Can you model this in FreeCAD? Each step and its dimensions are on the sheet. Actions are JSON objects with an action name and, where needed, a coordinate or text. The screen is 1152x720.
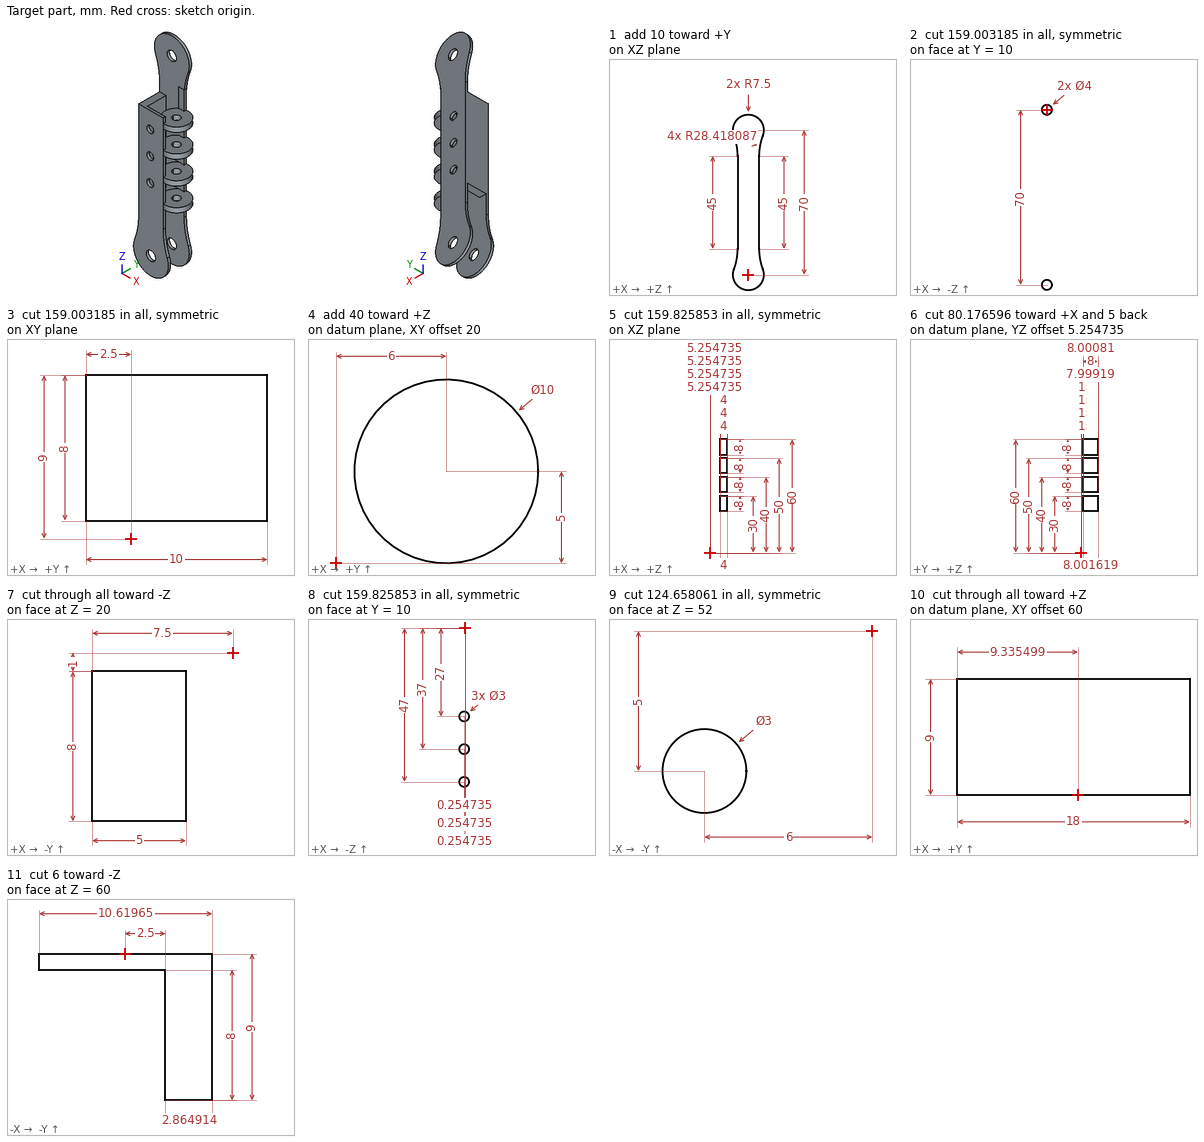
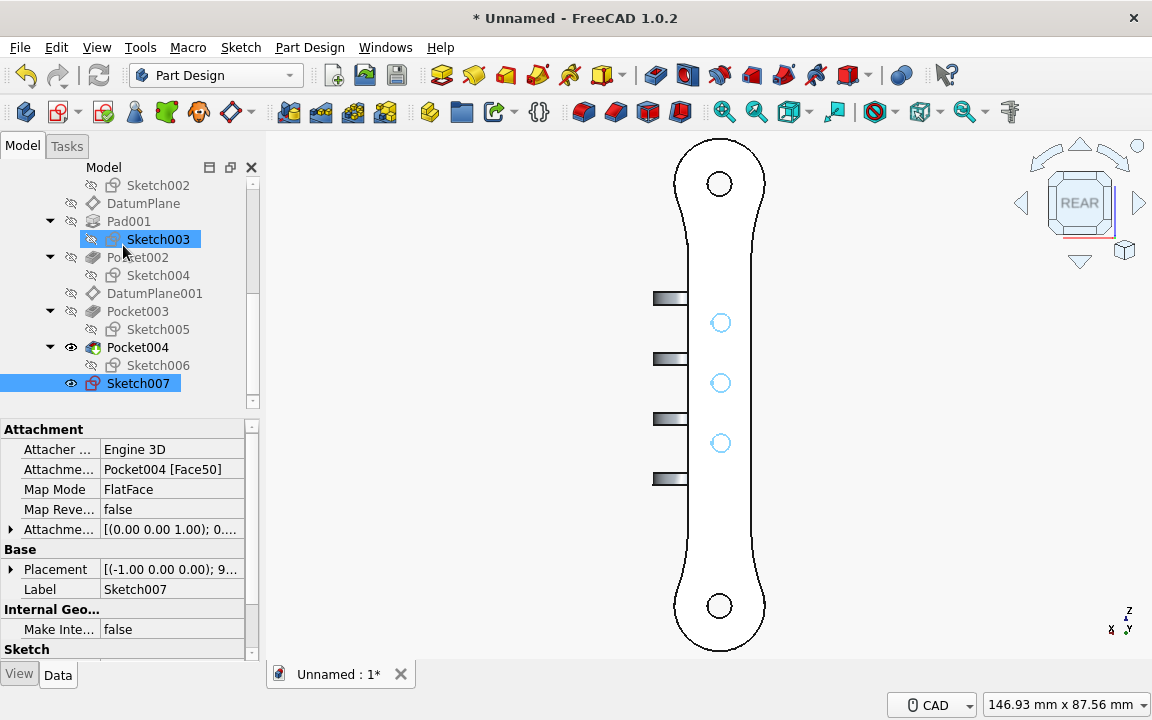
{"action": "left_click", "coordinate": [656, 76]}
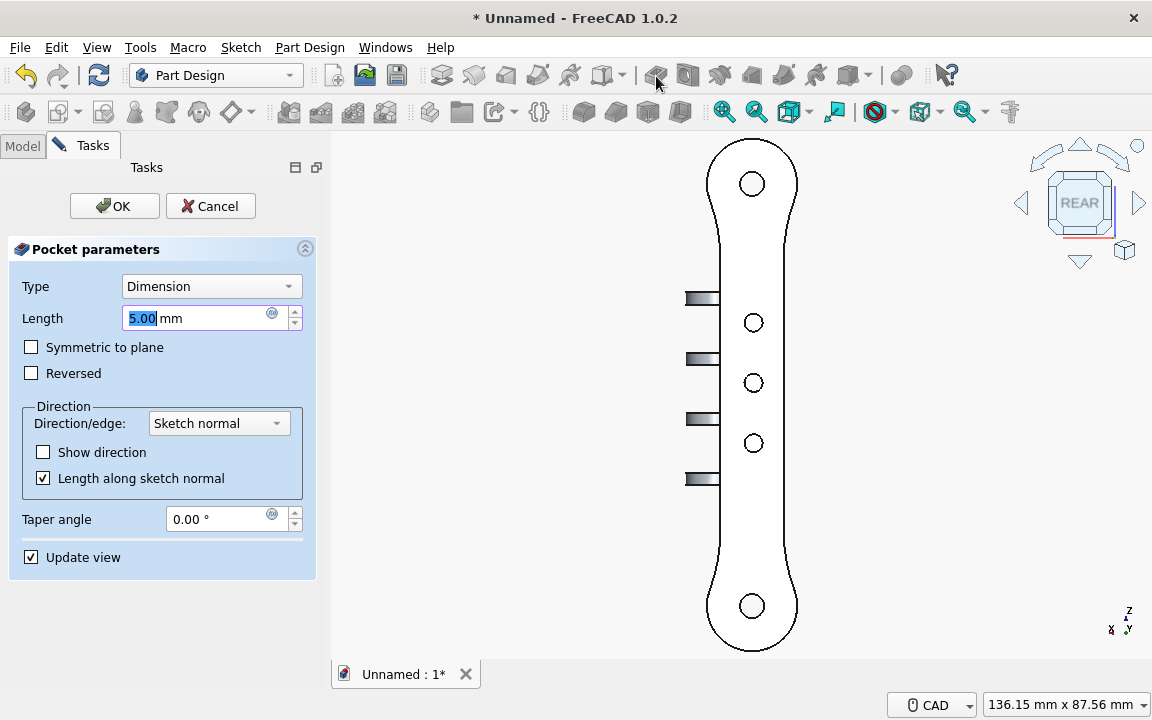
{"action": "type", "text": "159.825853"}
{"action": "key", "text": "Tab"}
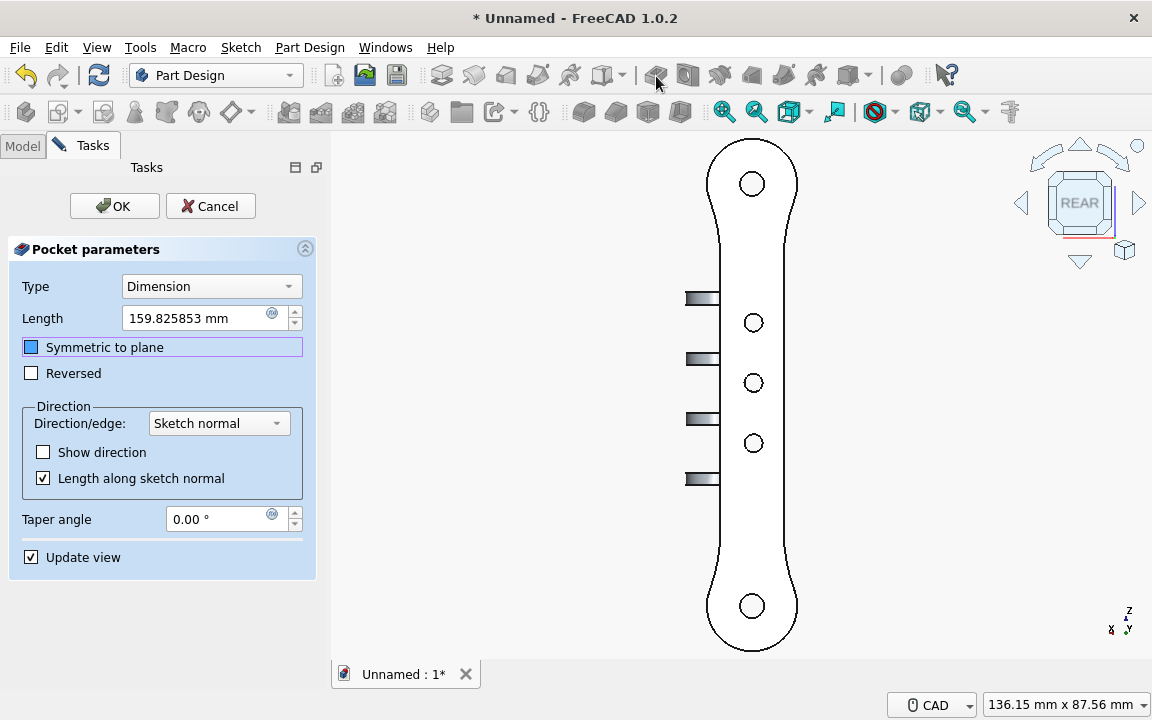
{"action": "left_click", "coordinate": [30, 347]}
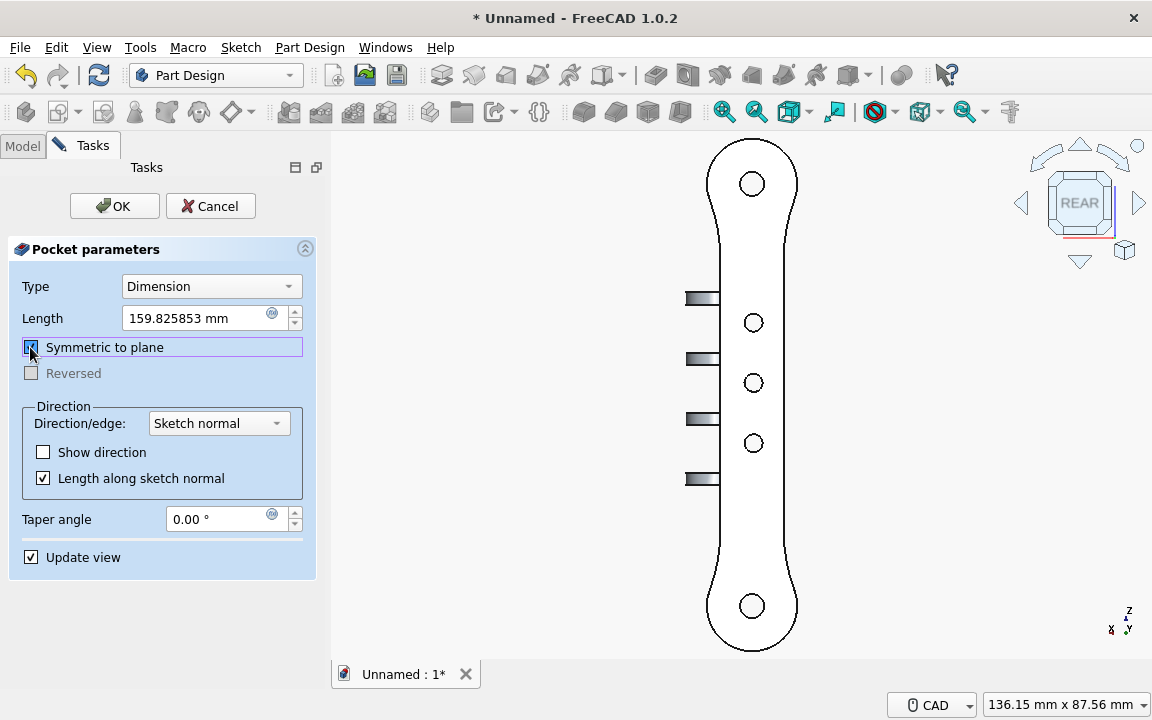
{"action": "left_click", "coordinate": [115, 206]}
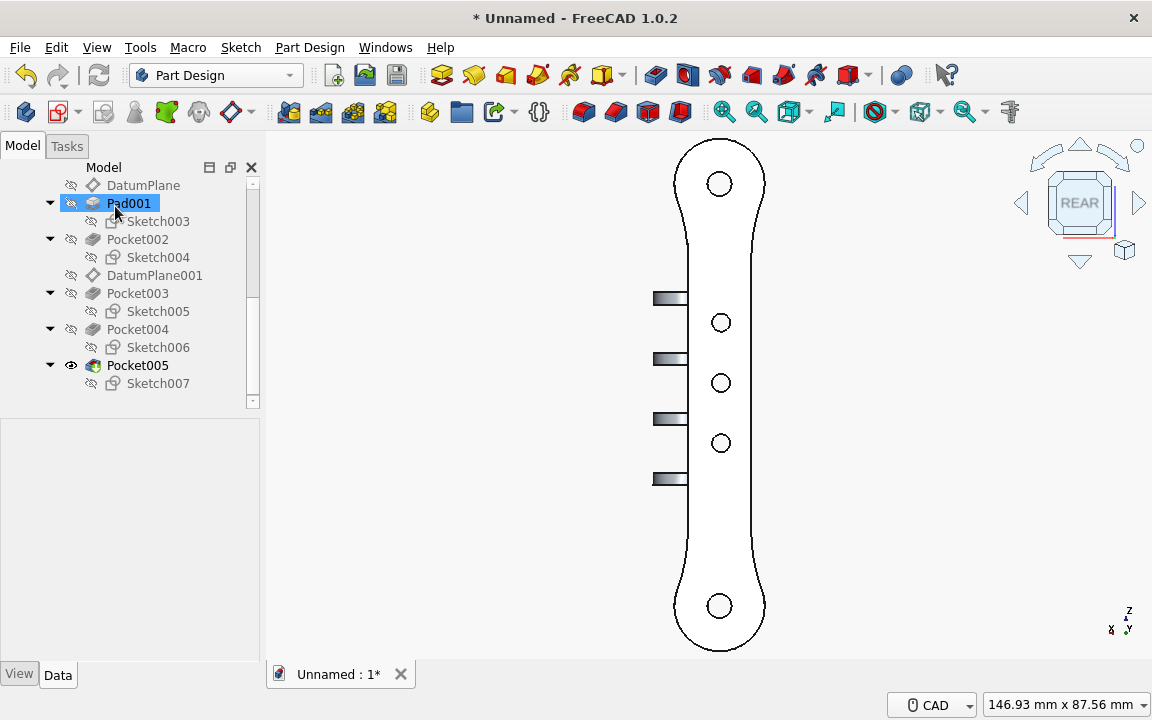
{"action": "key", "text": "0"}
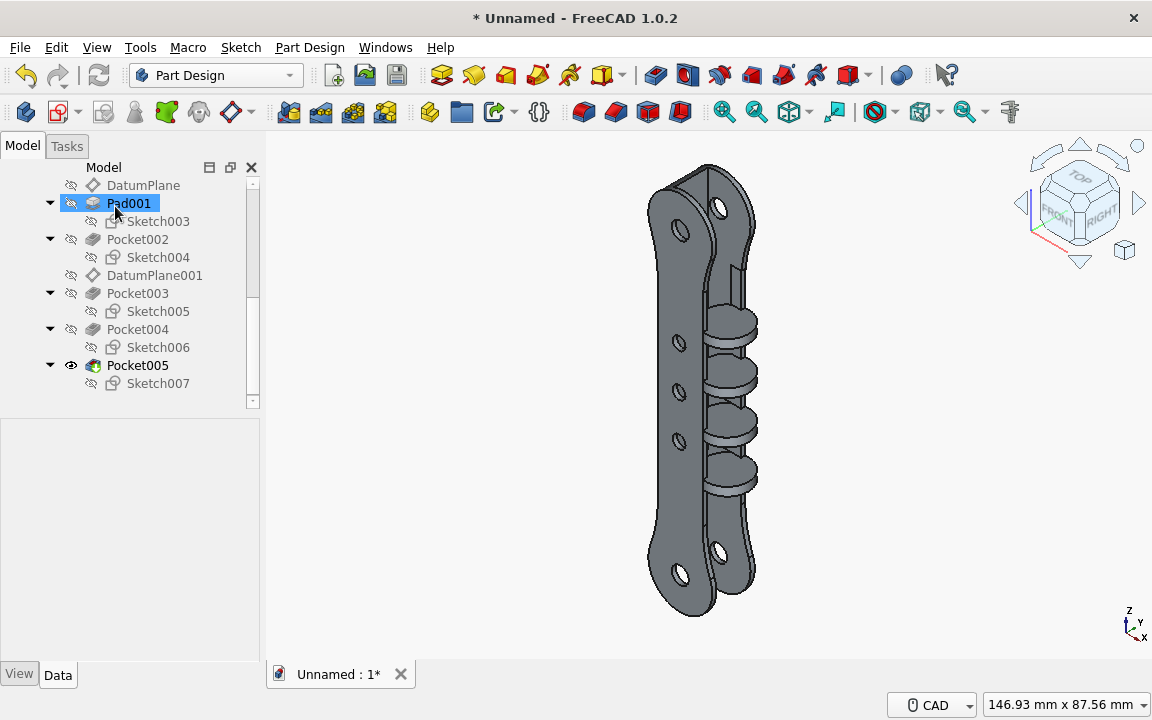
{"action": "left_click", "coordinate": [727, 321]}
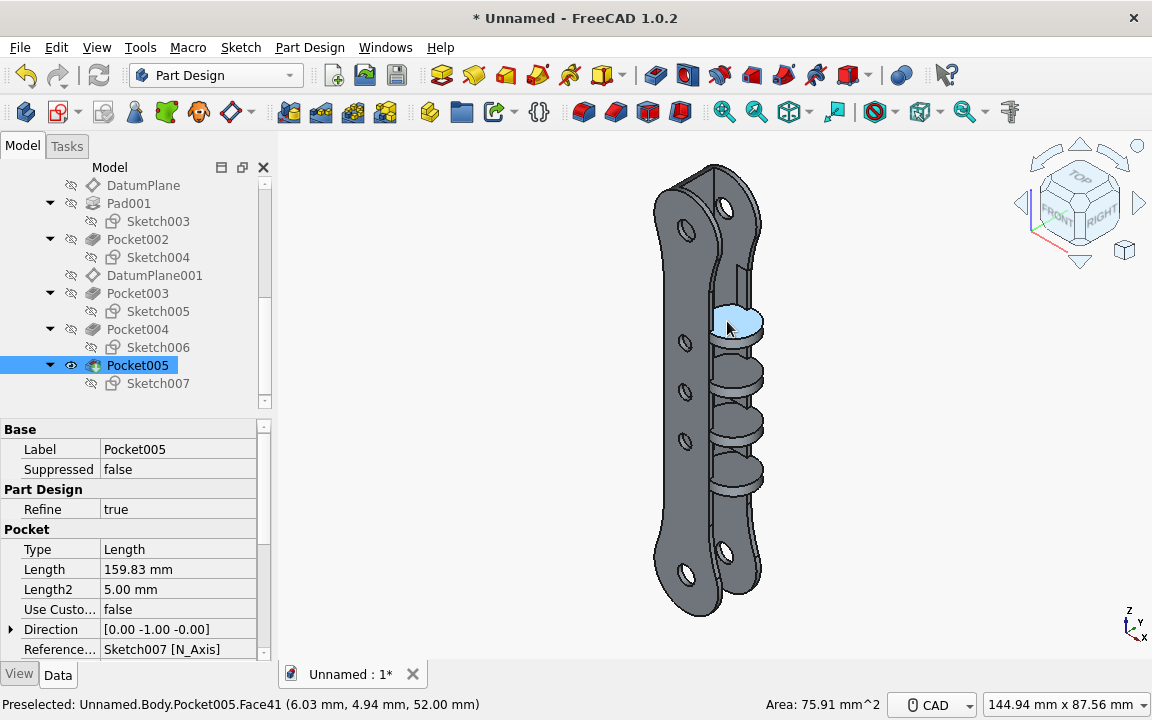
{"action": "left_click", "coordinate": [58, 112]}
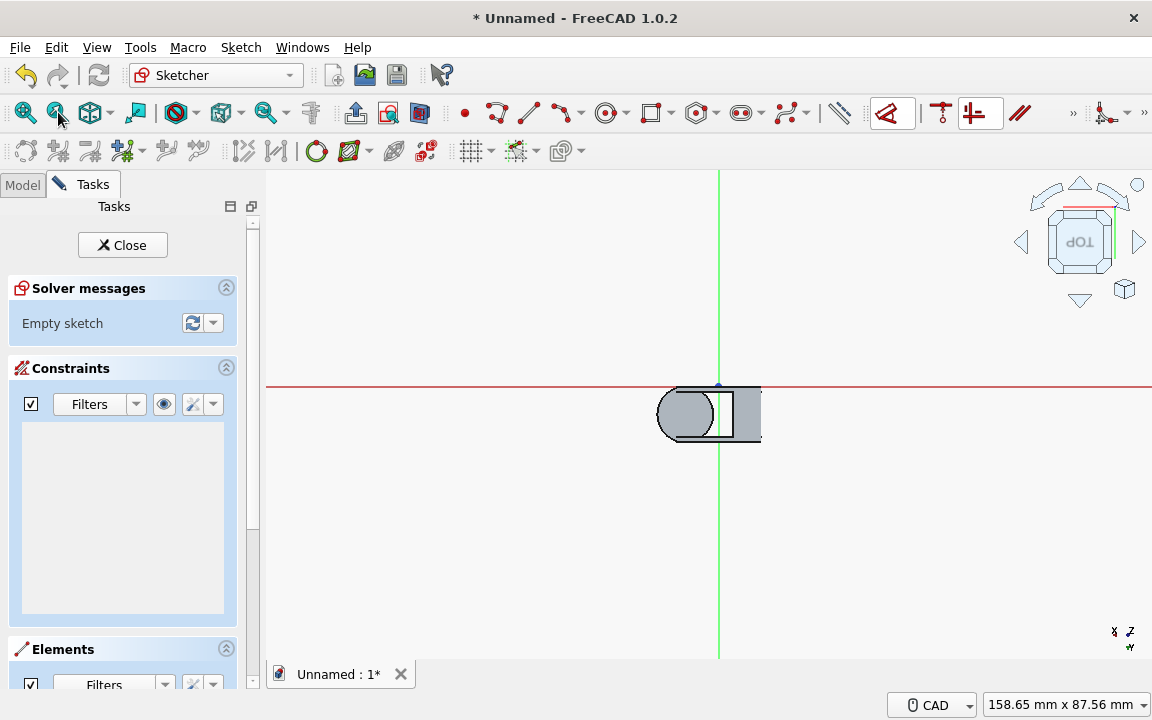
{"action": "scroll", "coordinate": [688, 415], "scroll_direction": "up", "scroll_amount": 15}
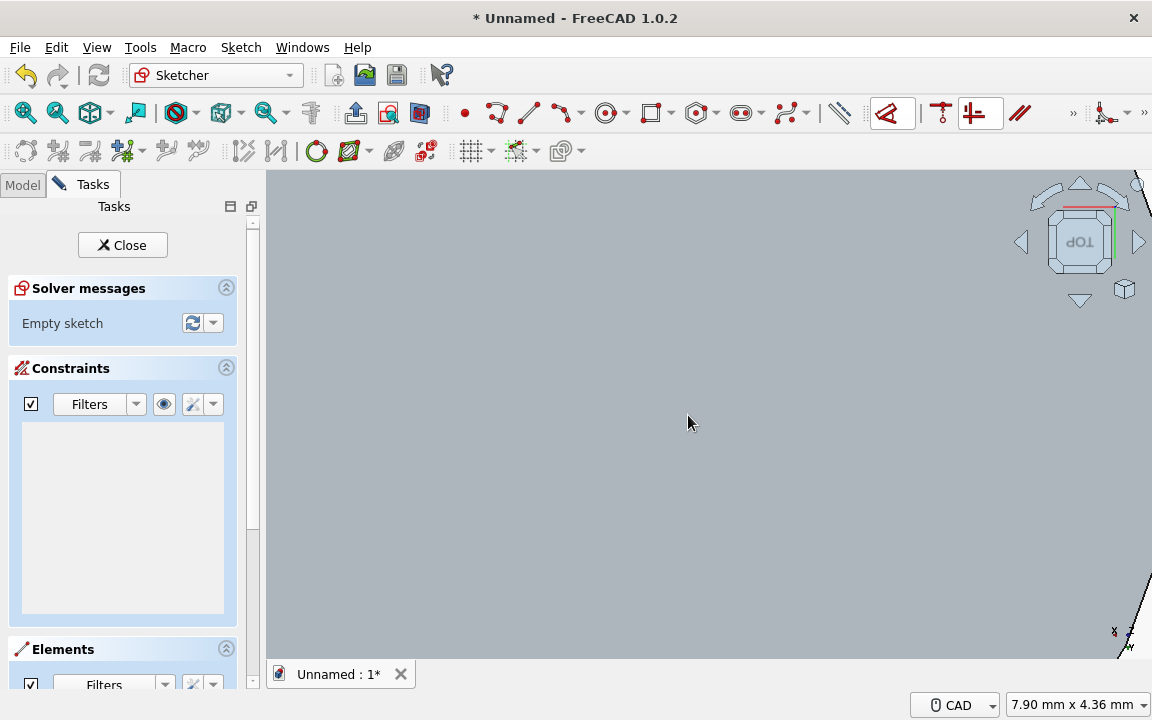
{"action": "left_click", "coordinate": [606, 114]}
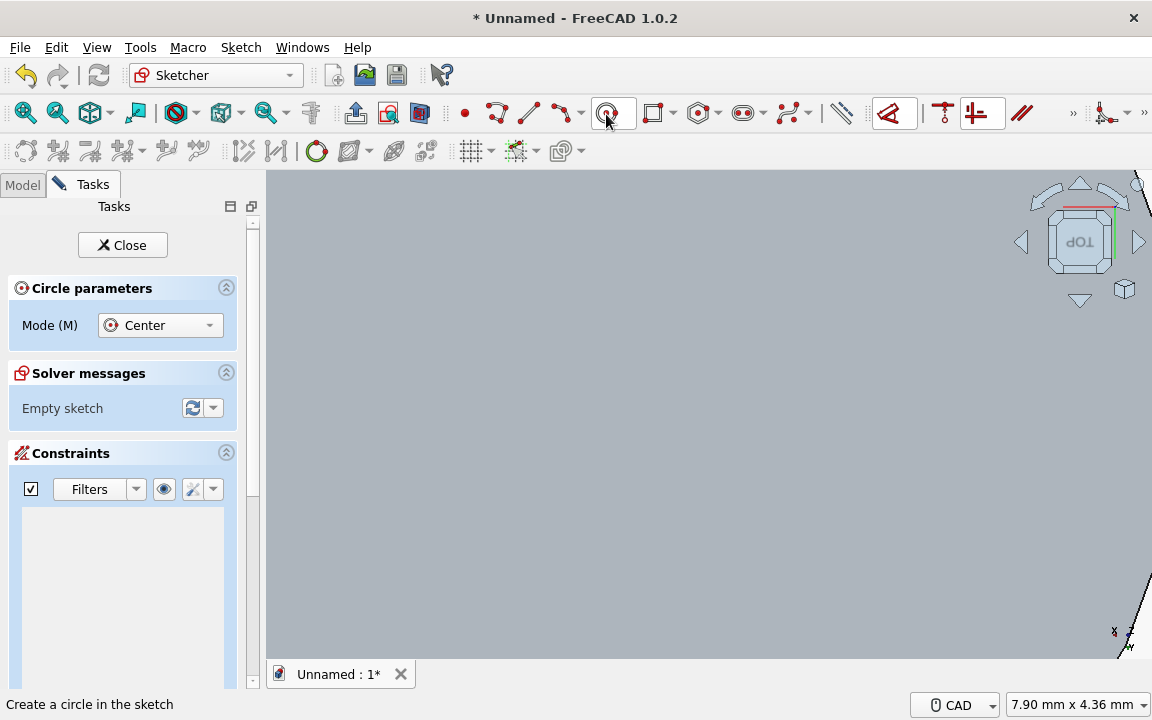
{"action": "left_click", "coordinate": [624, 395]}
{"action": "left_click", "coordinate": [743, 276]}
{"action": "key", "text": "Escape"}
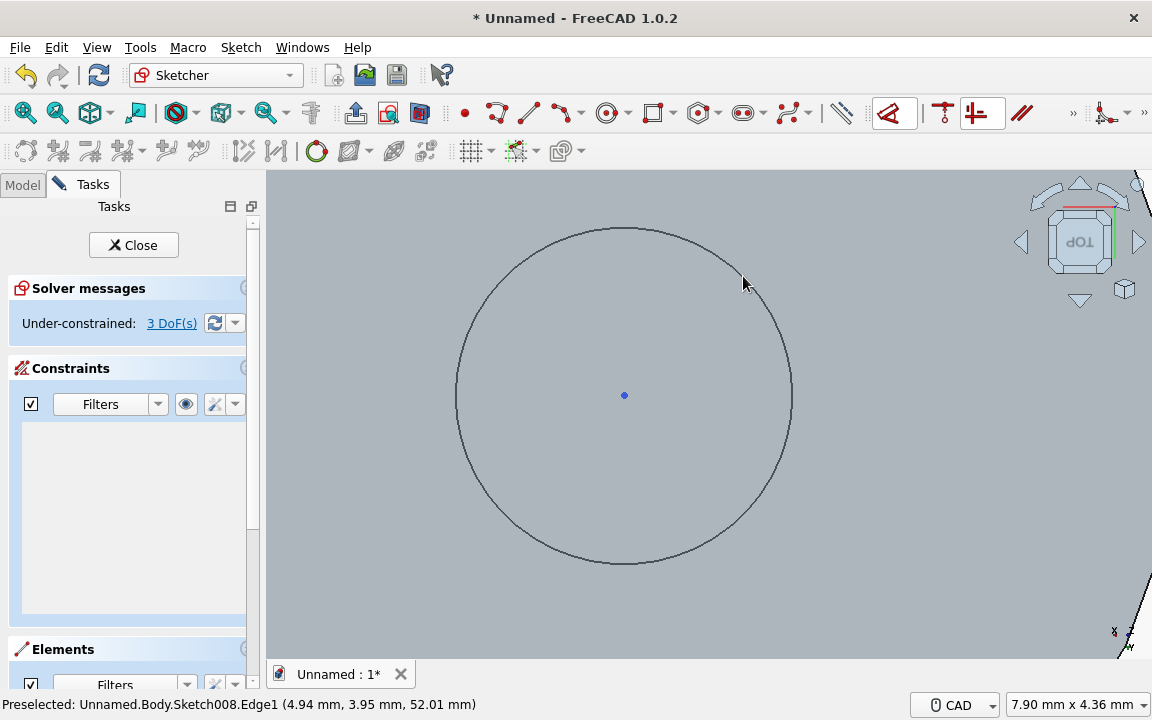
{"action": "left_click", "coordinate": [743, 277]}